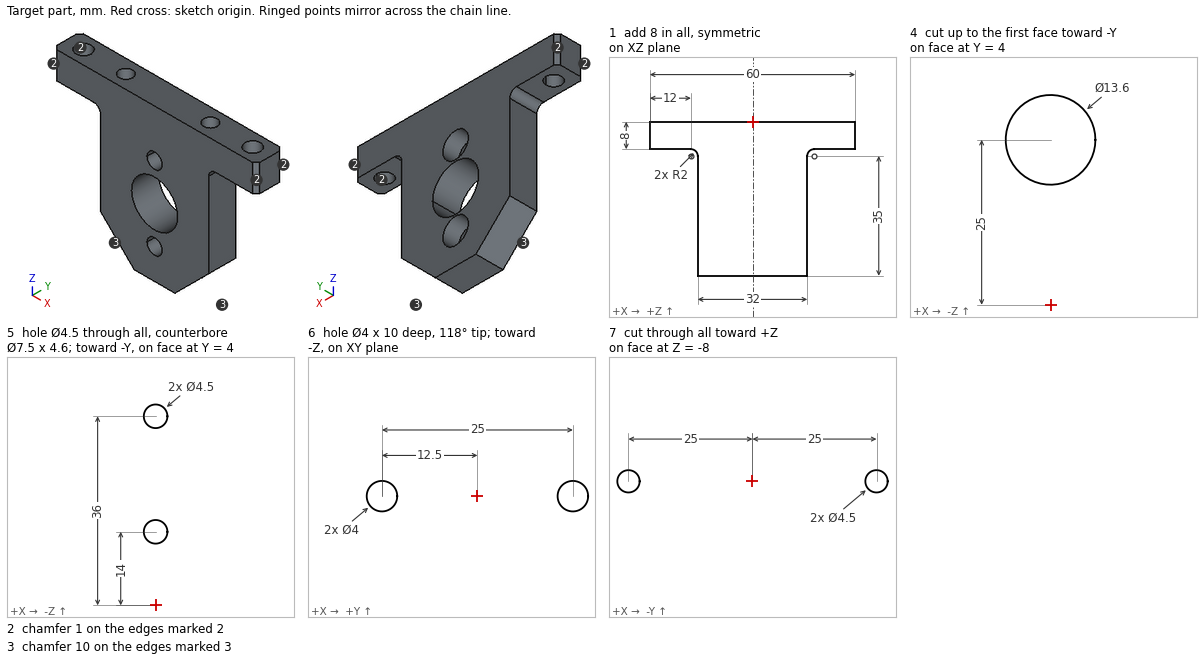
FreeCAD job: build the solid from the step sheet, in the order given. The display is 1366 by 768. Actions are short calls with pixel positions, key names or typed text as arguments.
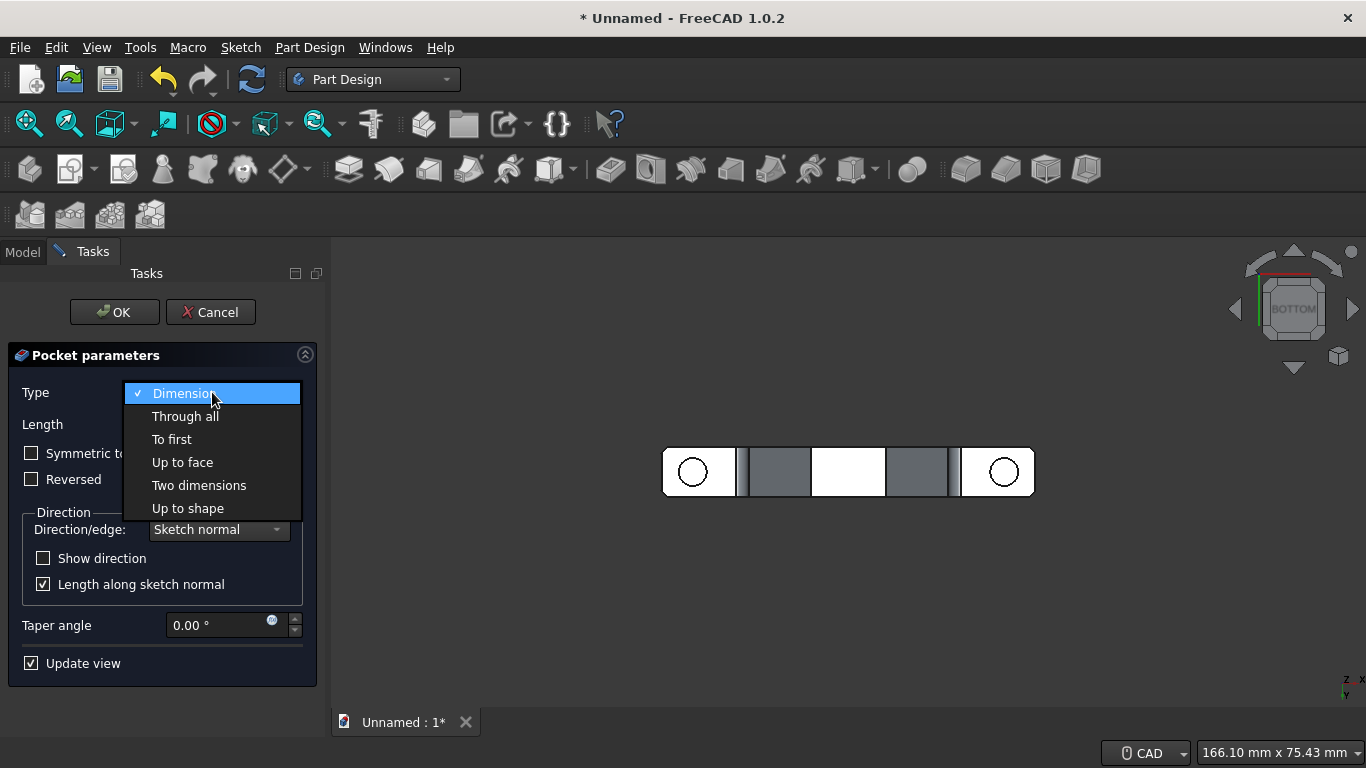
click(212, 416)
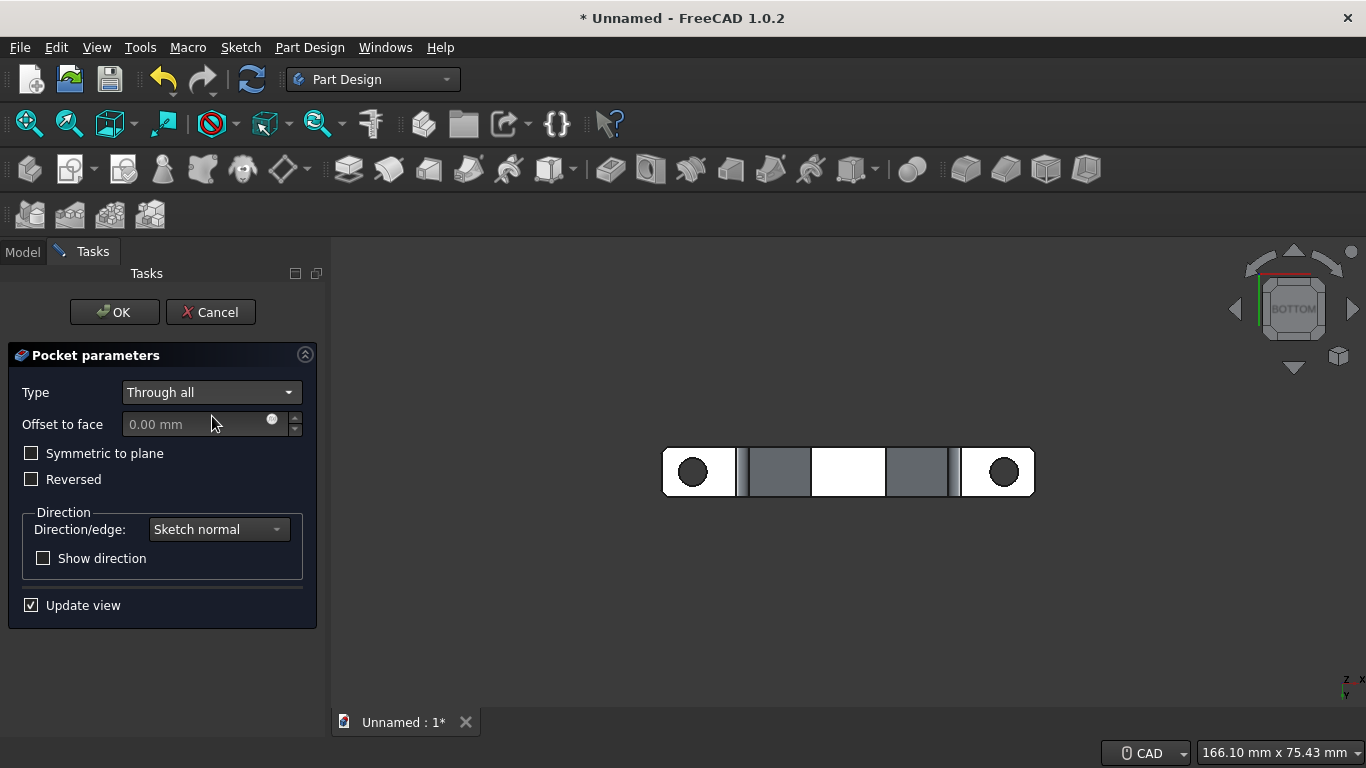
click(115, 312)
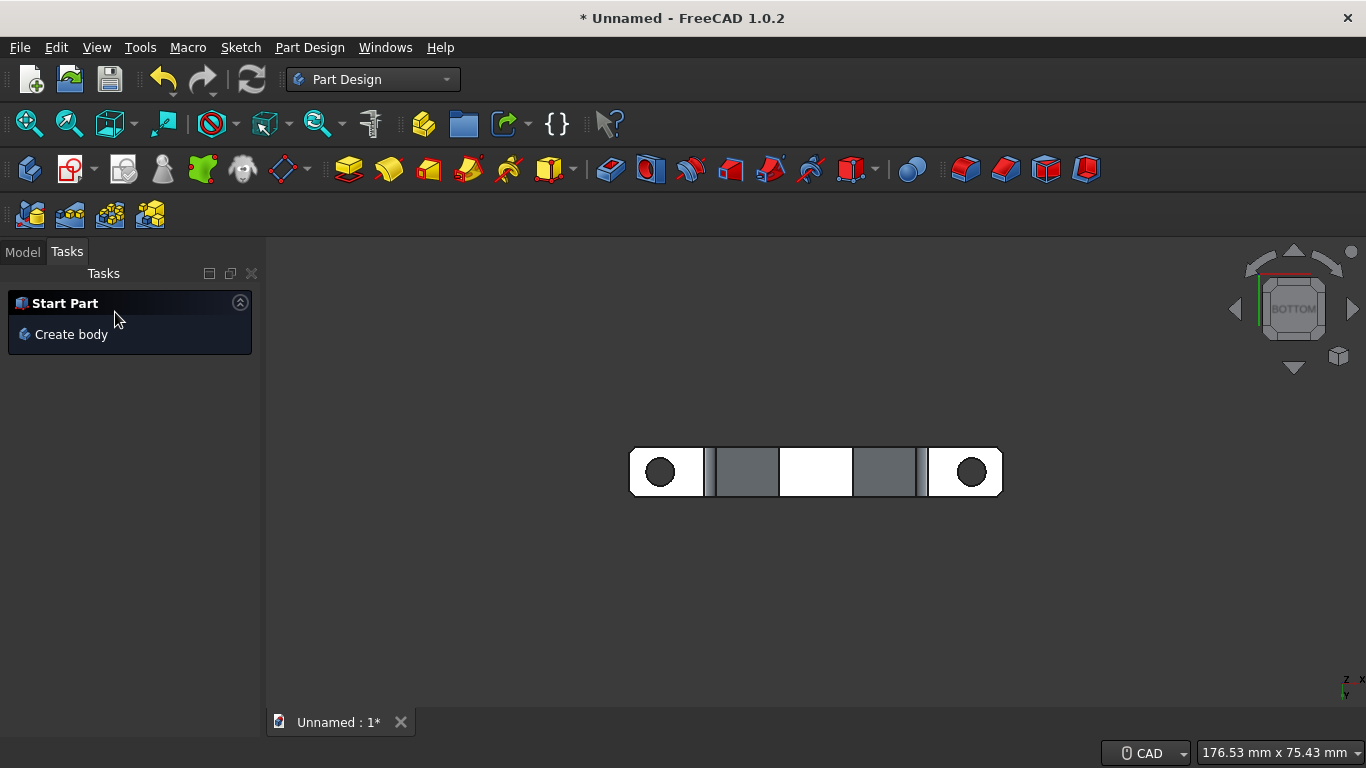
key(0)